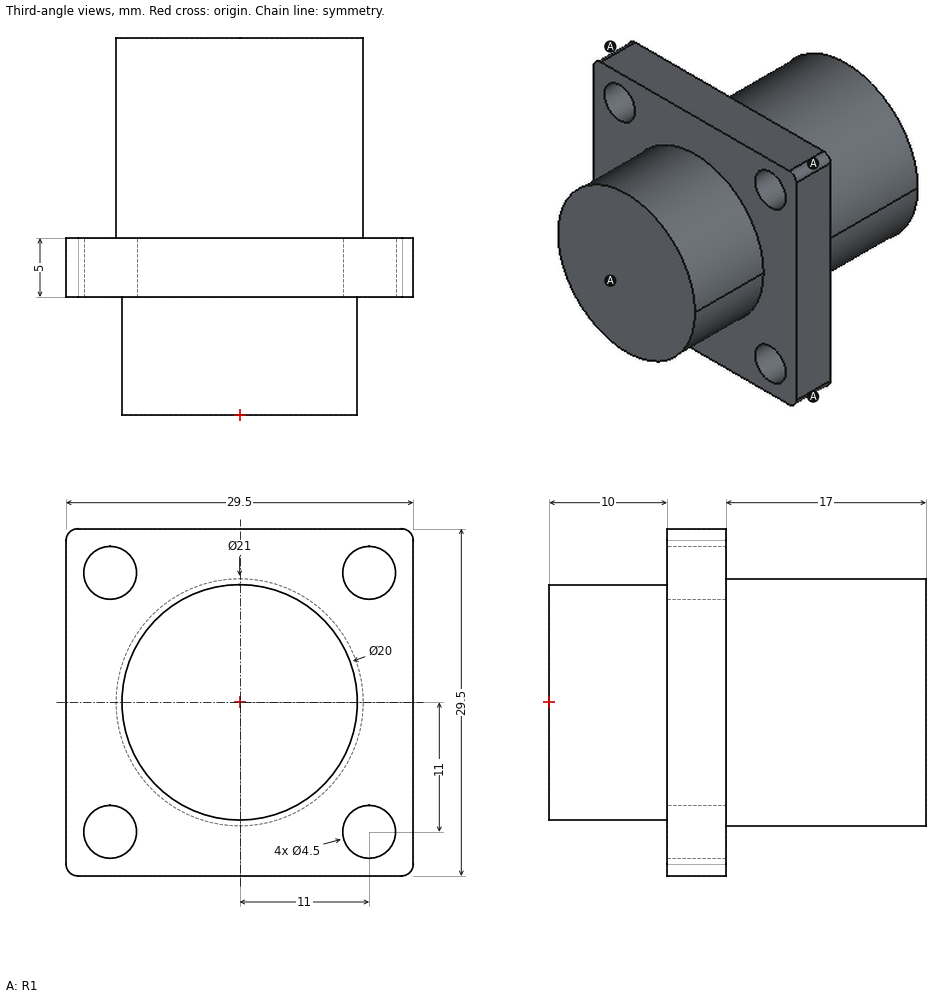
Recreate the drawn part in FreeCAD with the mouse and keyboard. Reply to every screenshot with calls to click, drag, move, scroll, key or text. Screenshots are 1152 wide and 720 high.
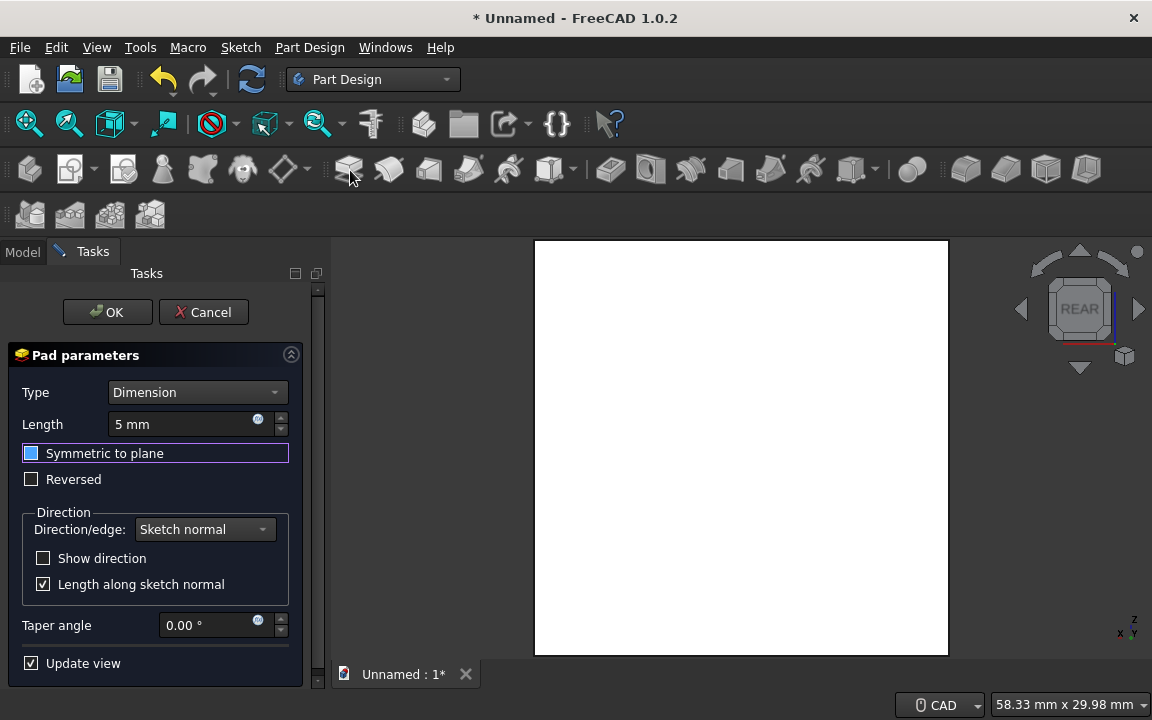
click(108, 312)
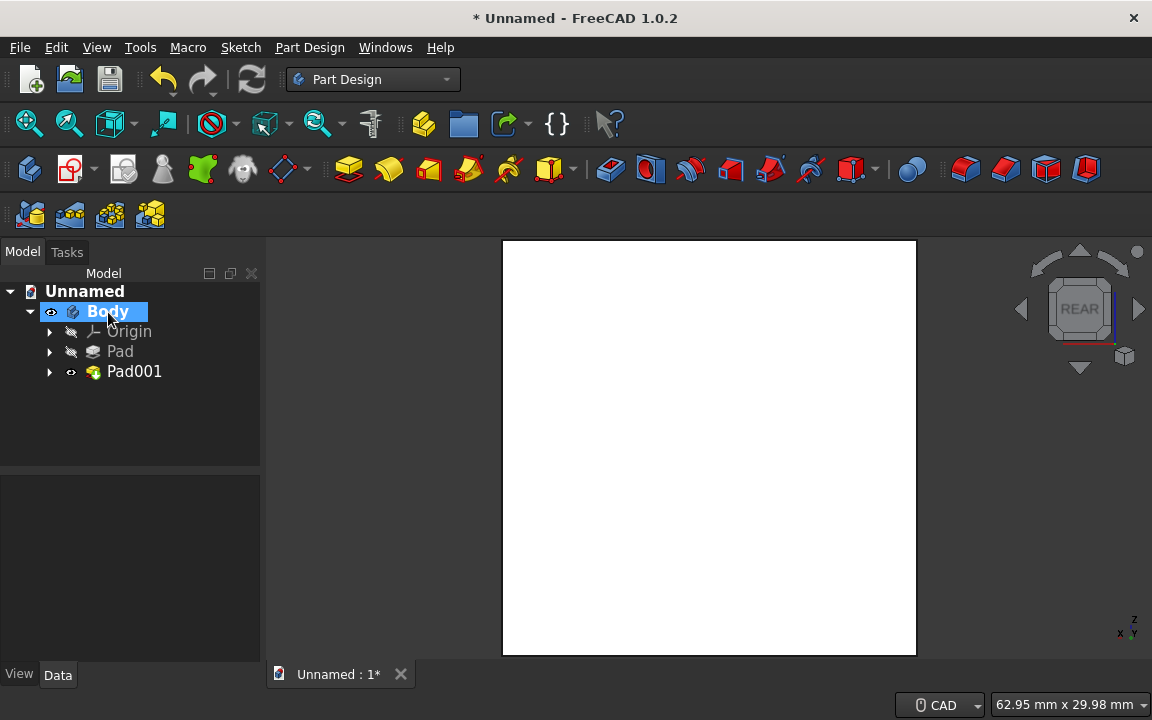
click(709, 447)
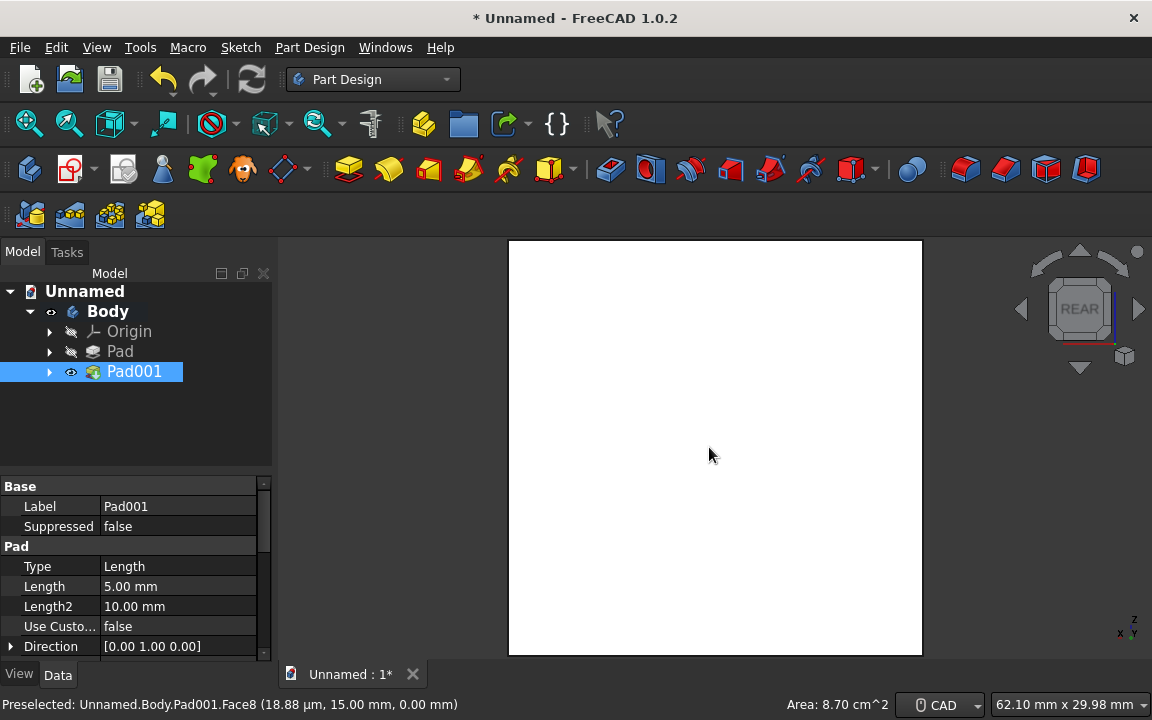
click(70, 170)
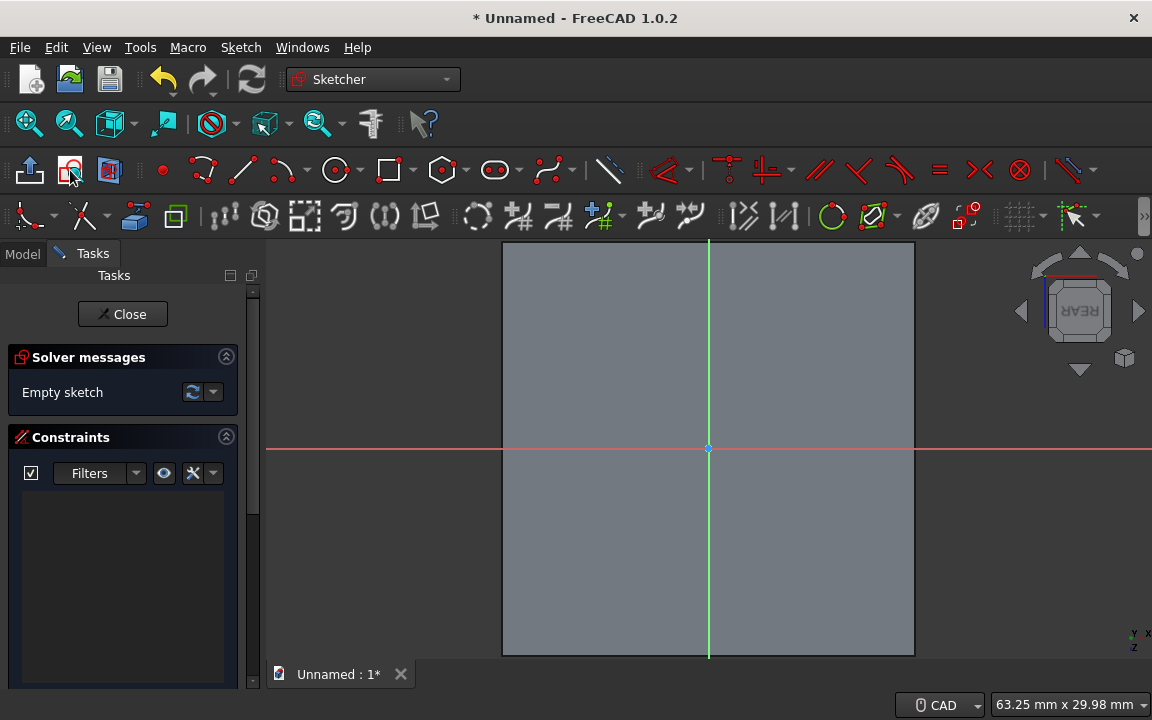
key(g)
key(c)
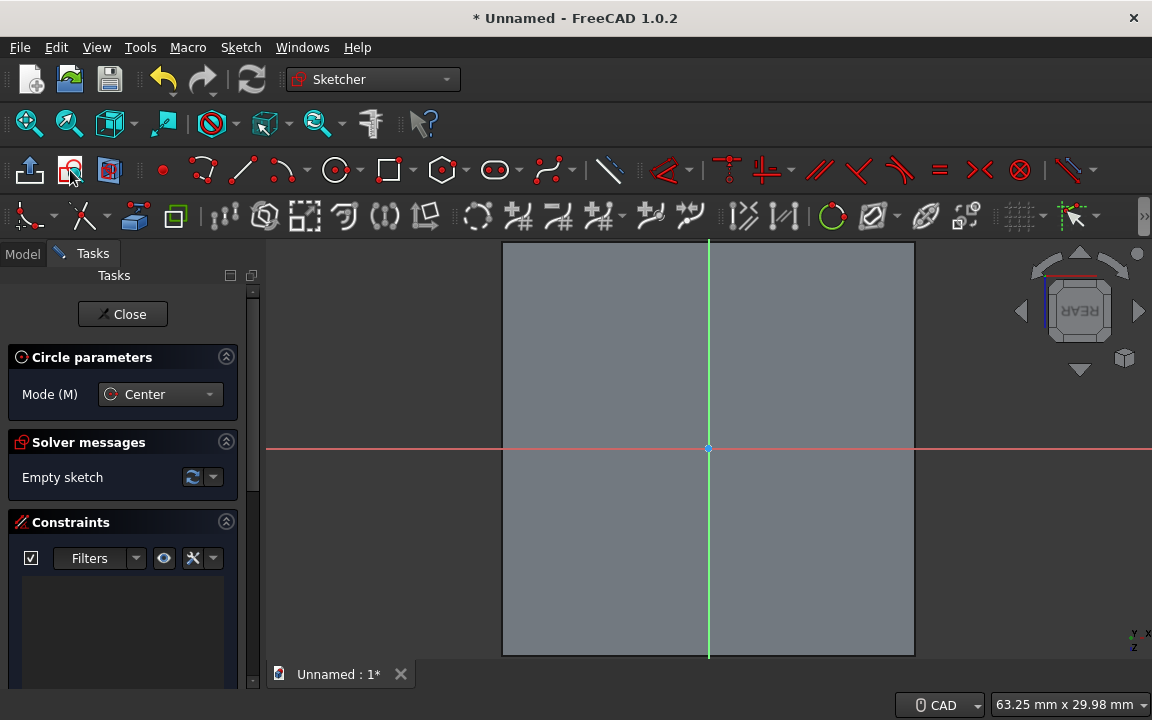
click(709, 449)
move(813, 345)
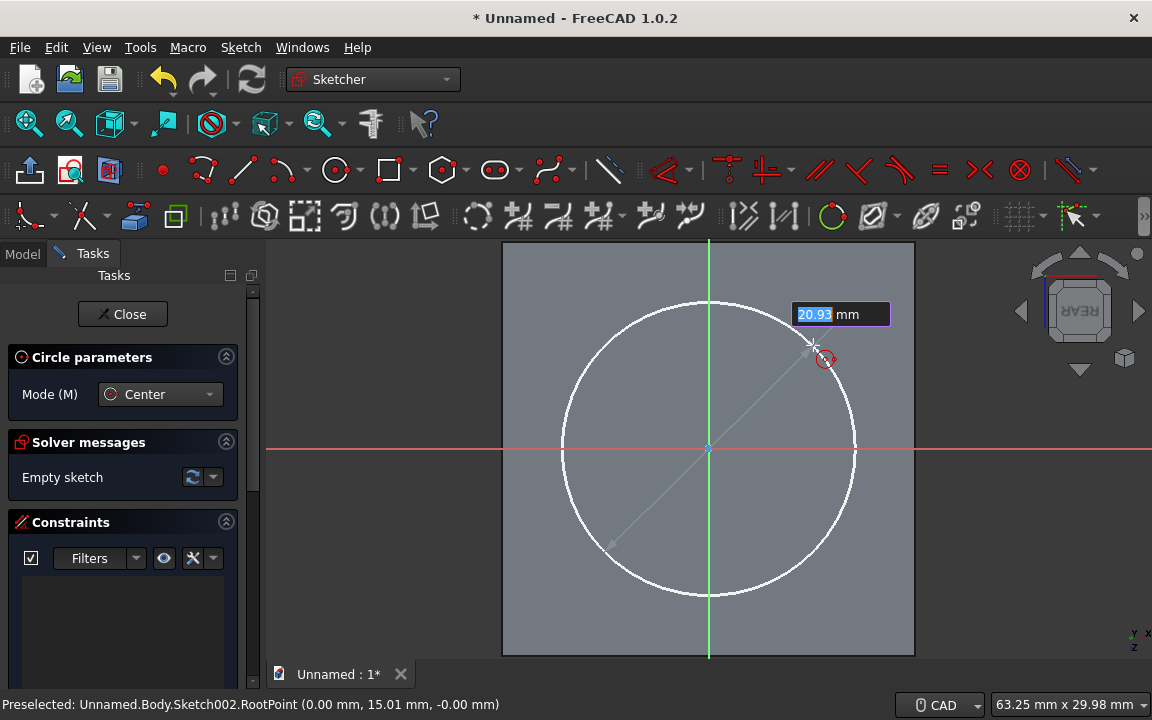
text(21)
key(Return)
key(Escape)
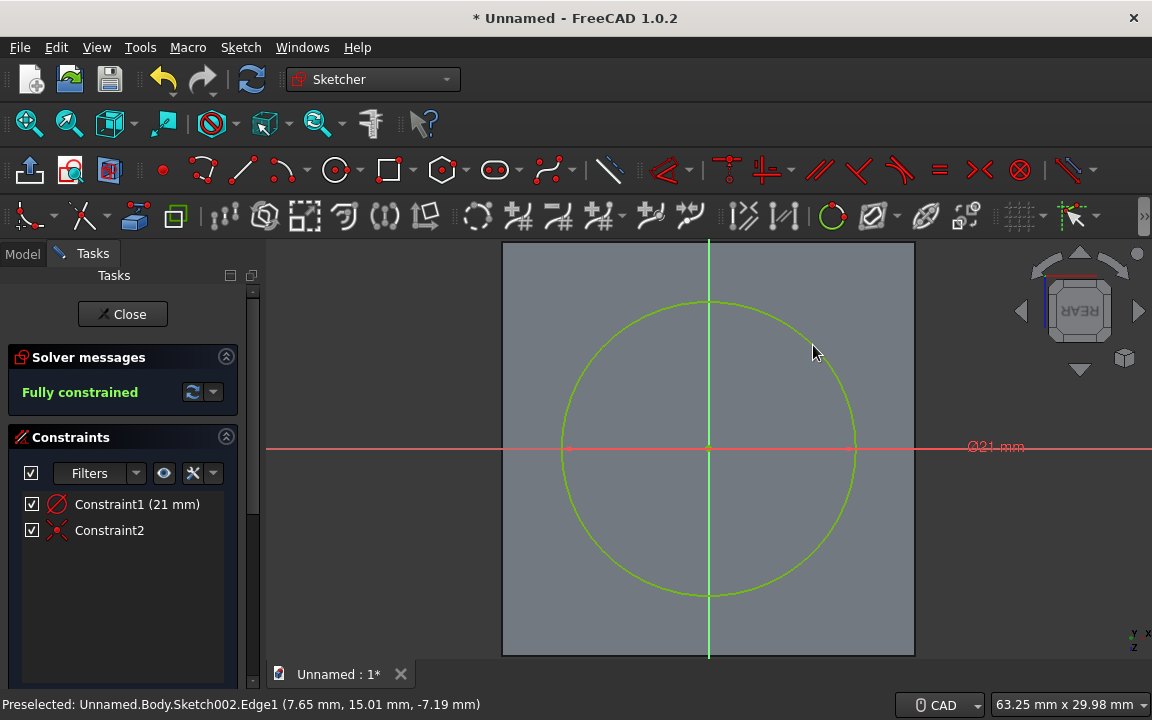
click(123, 314)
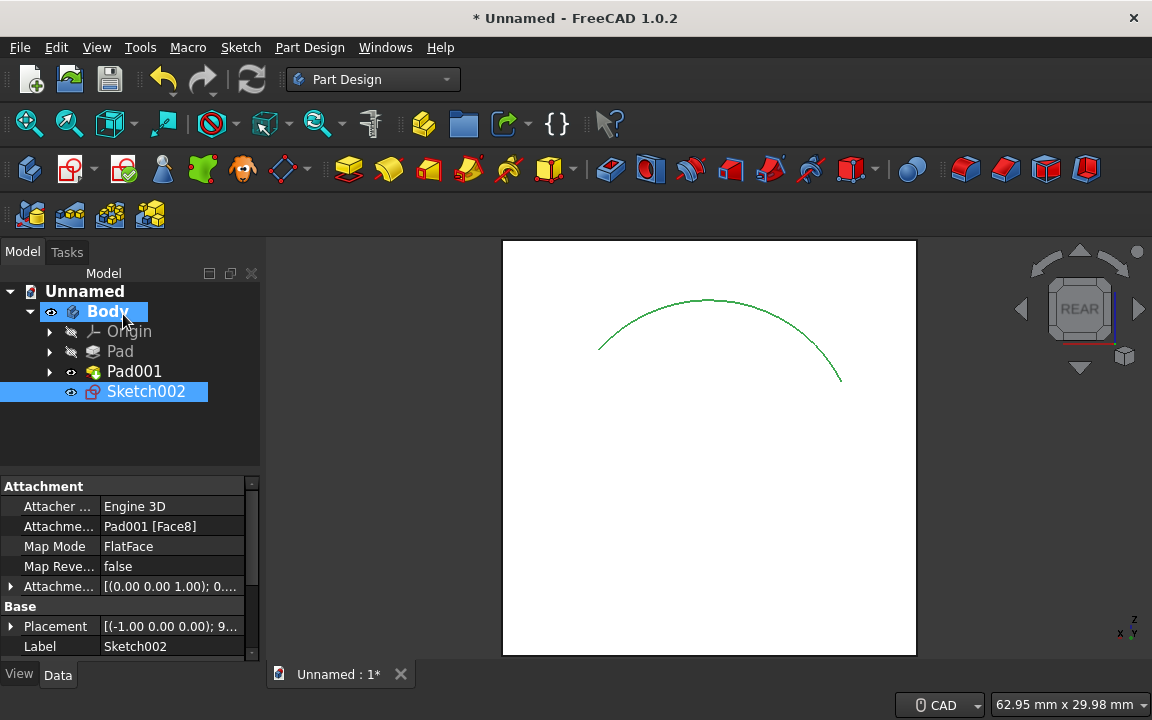
click(350, 170)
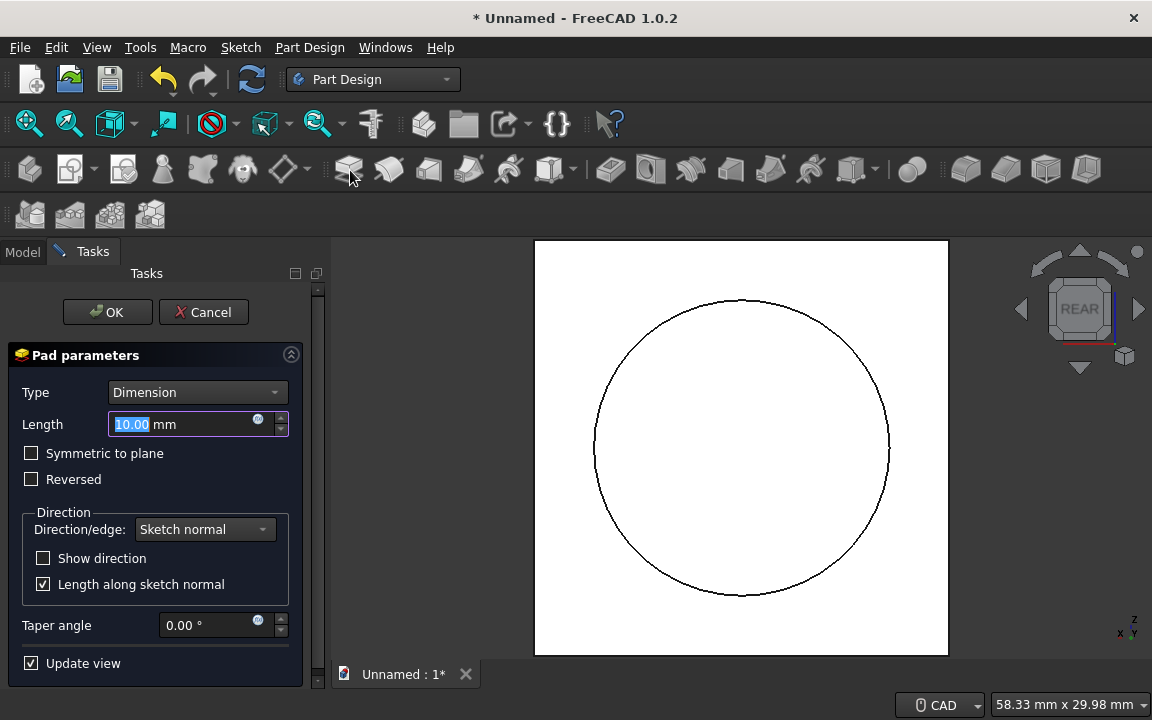
text(17)
key(Tab)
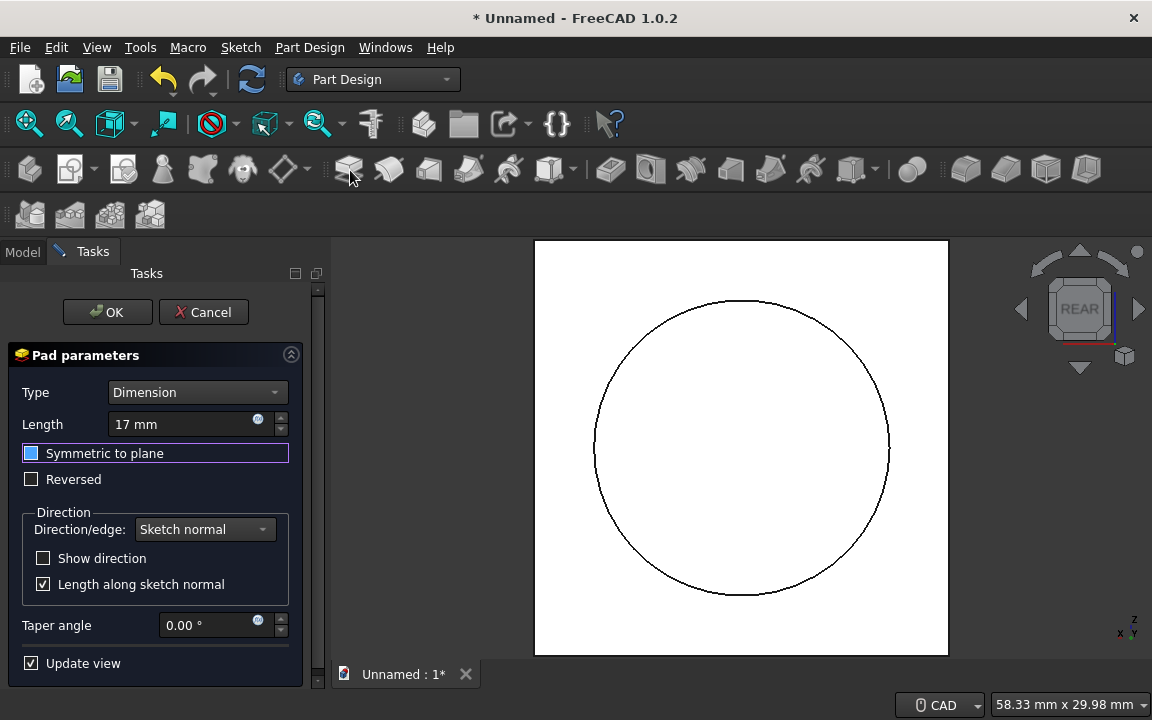
click(108, 312)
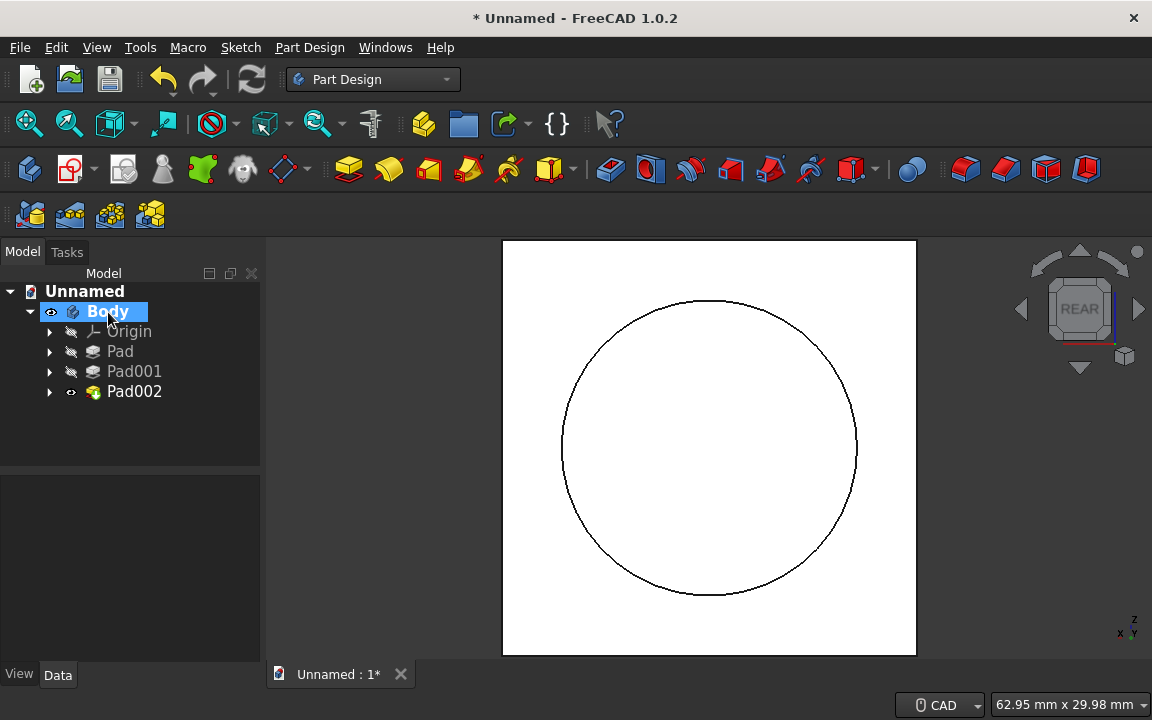
click(531, 625)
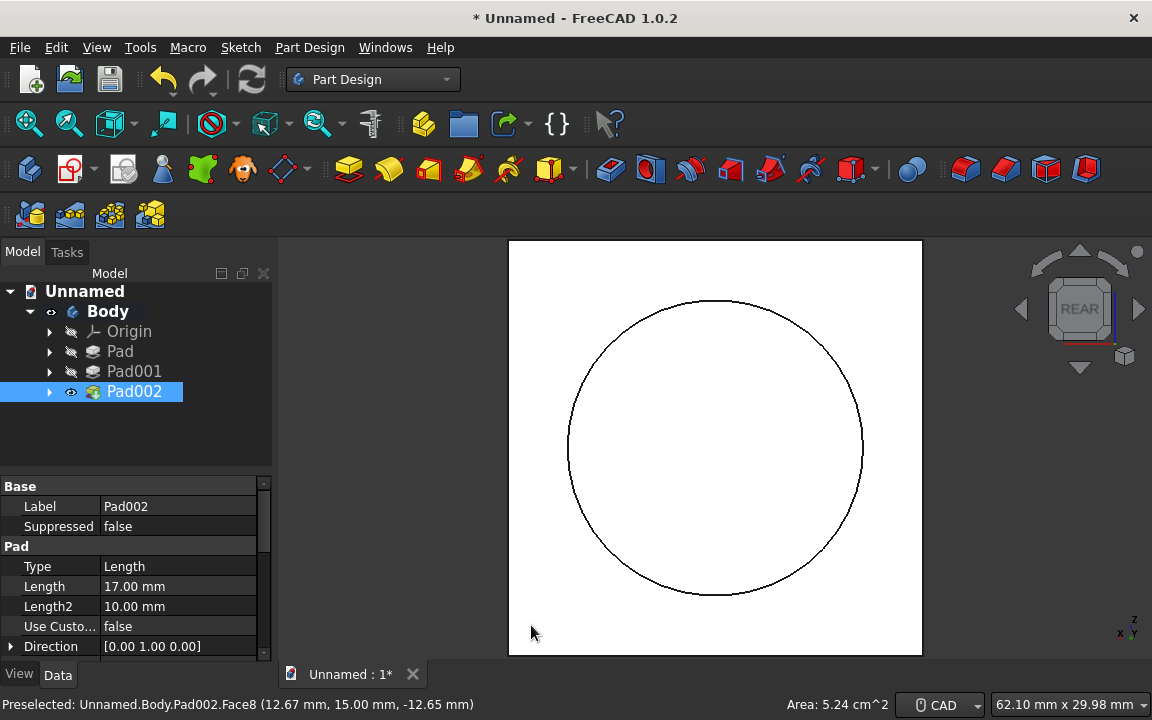
click(70, 170)